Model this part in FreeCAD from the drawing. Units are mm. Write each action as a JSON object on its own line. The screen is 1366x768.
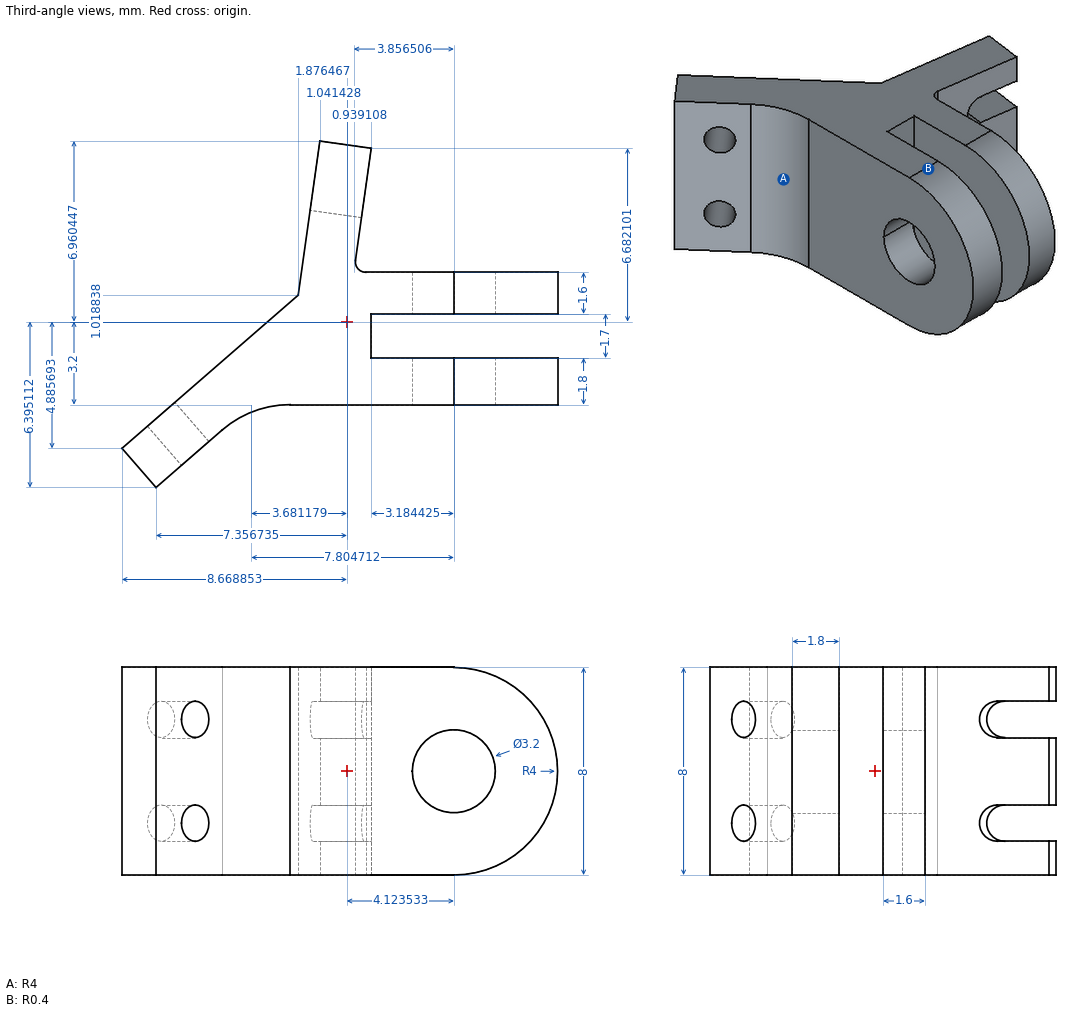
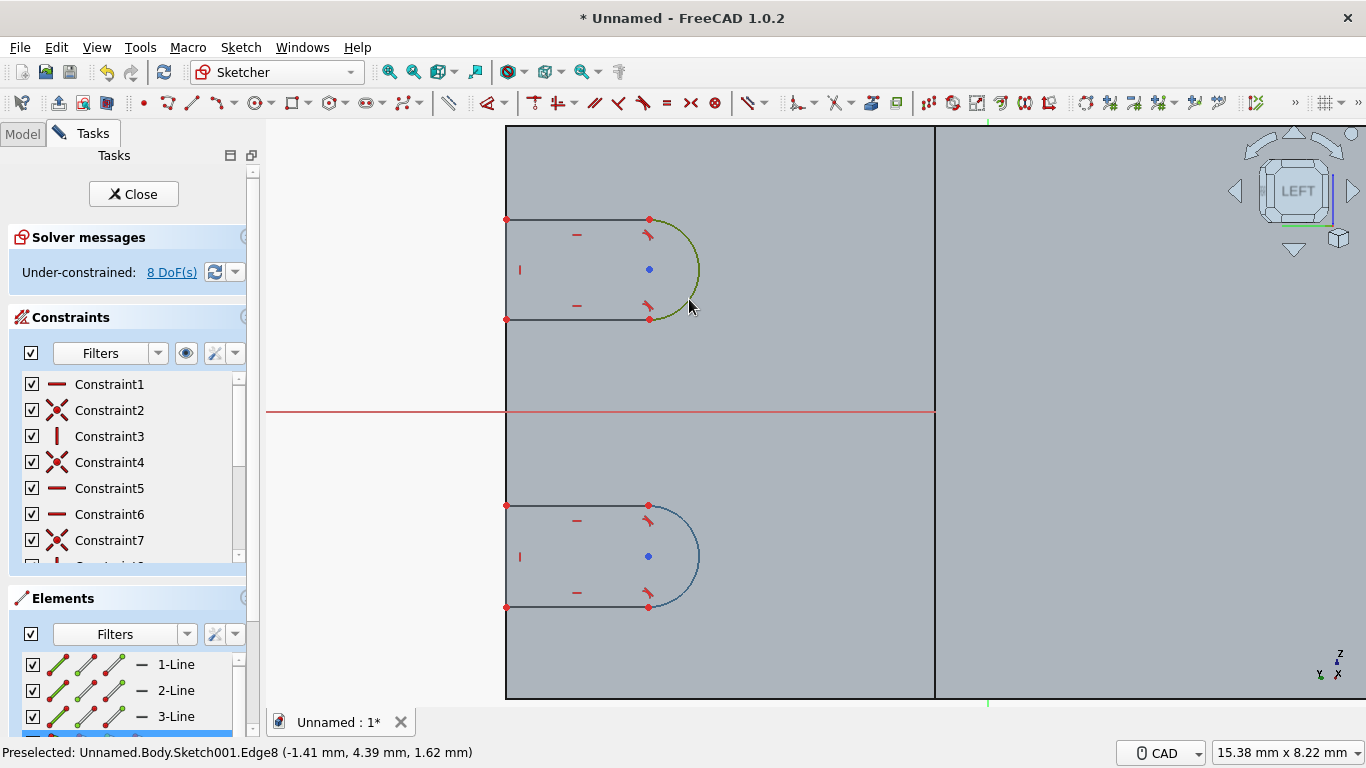
{"action": "left_click", "coordinate": [668, 104]}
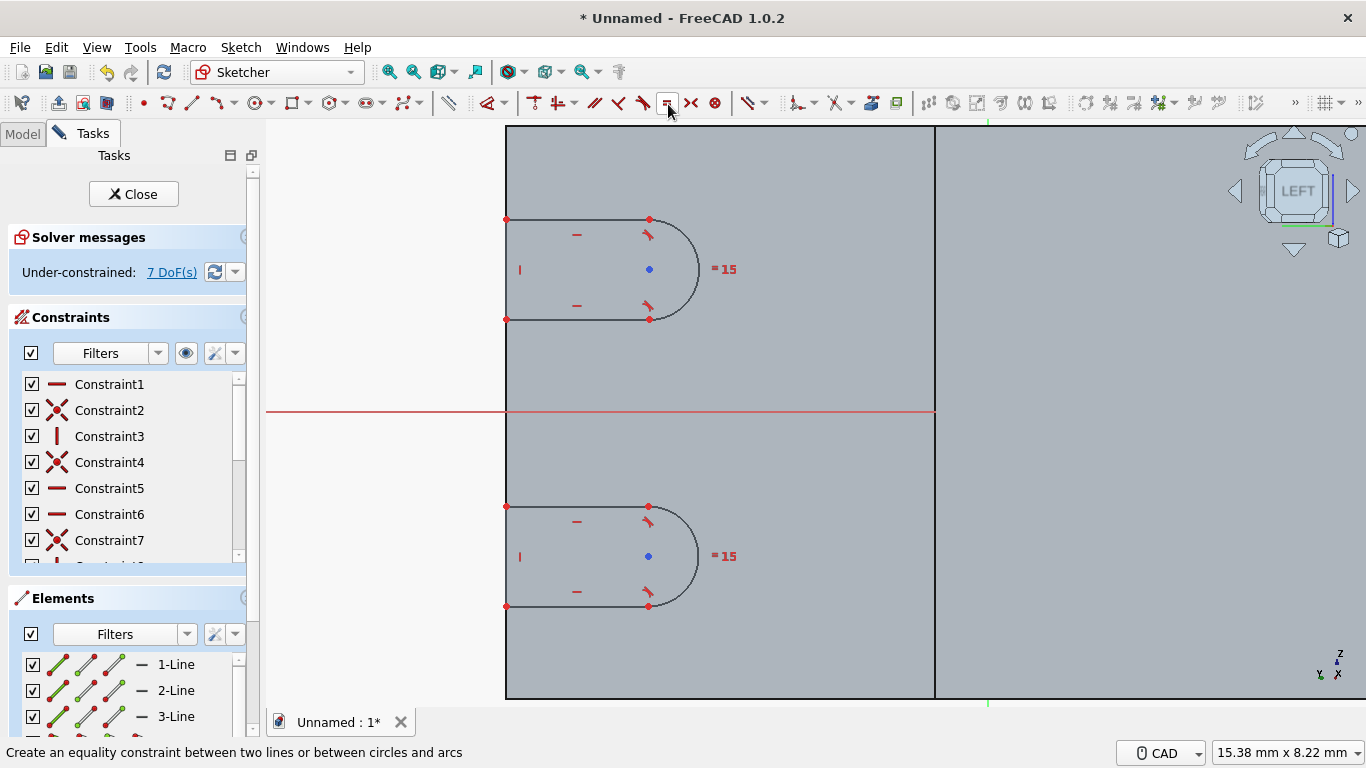
{"action": "left_click", "coordinate": [649, 557]}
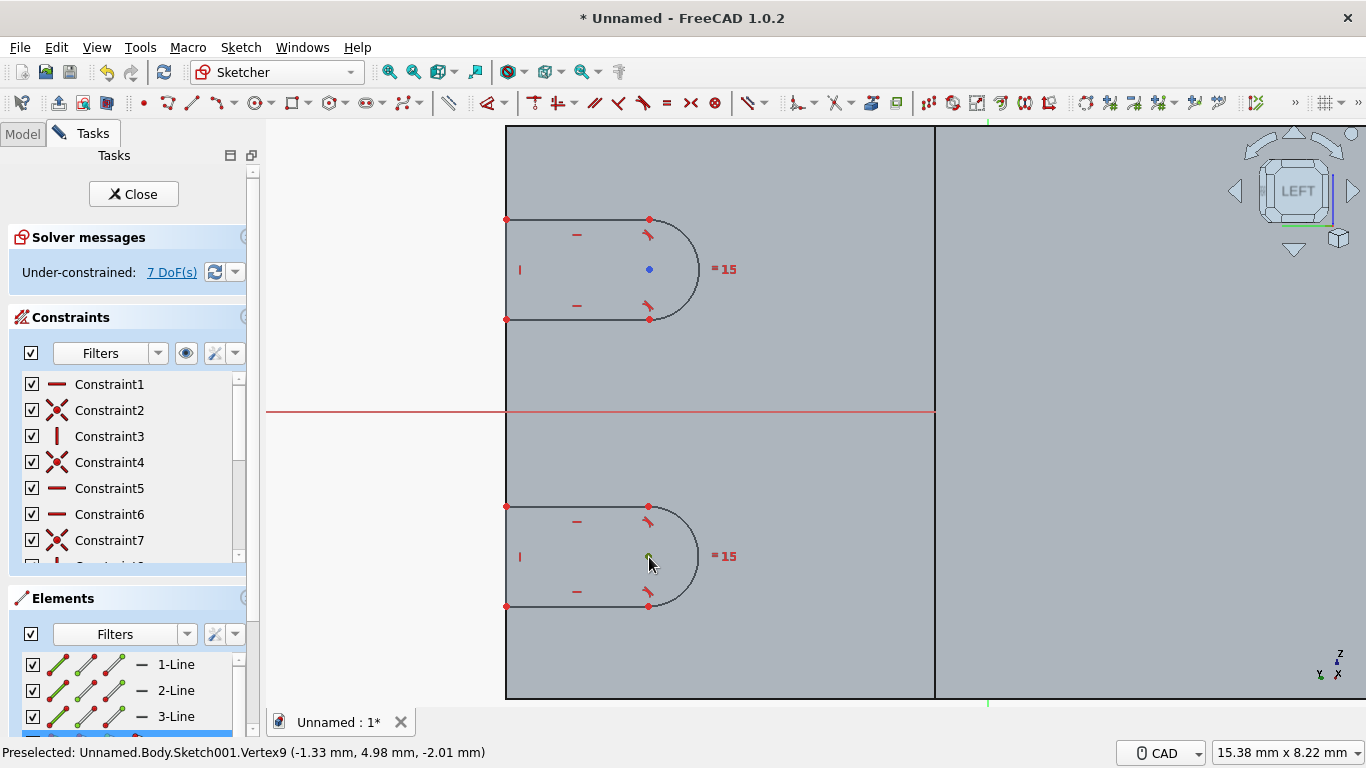
{"action": "left_click", "coordinate": [649, 270]}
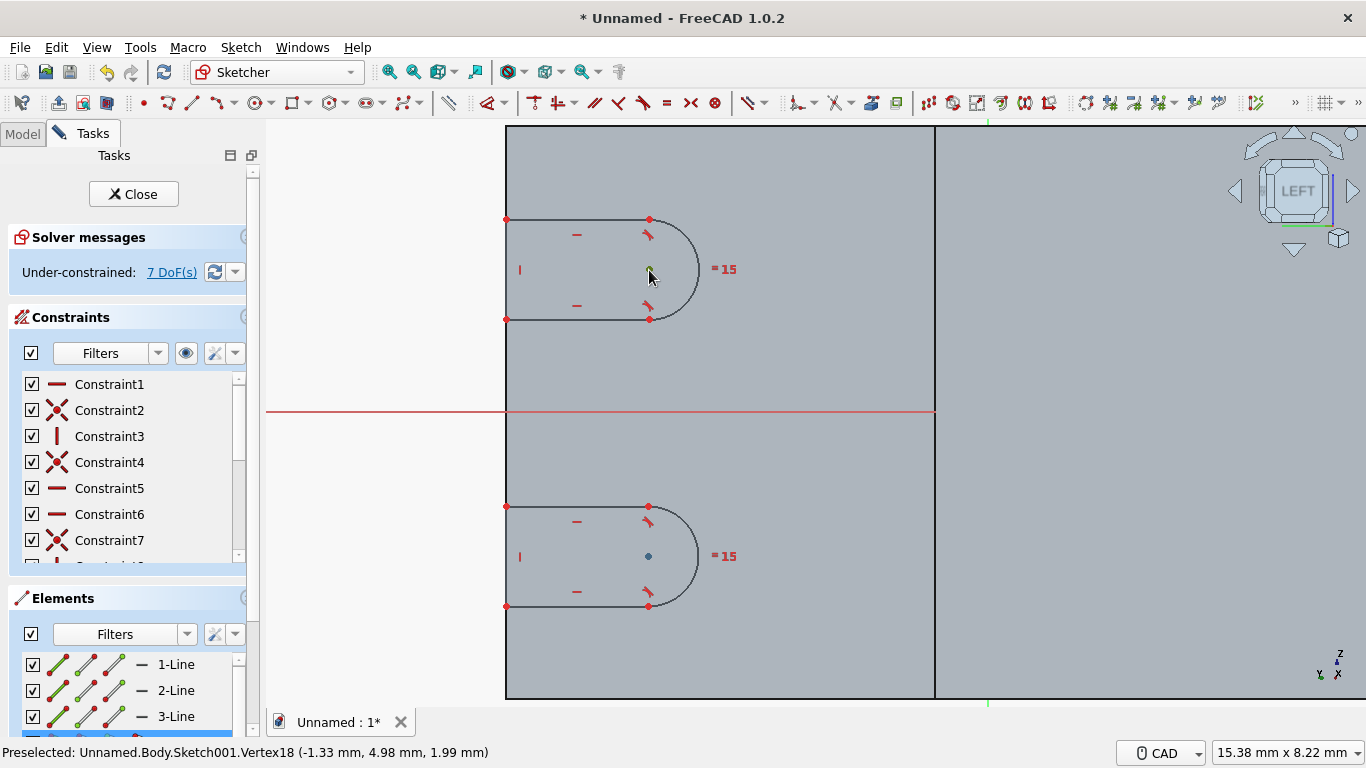
{"action": "left_click", "coordinate": [359, 412]}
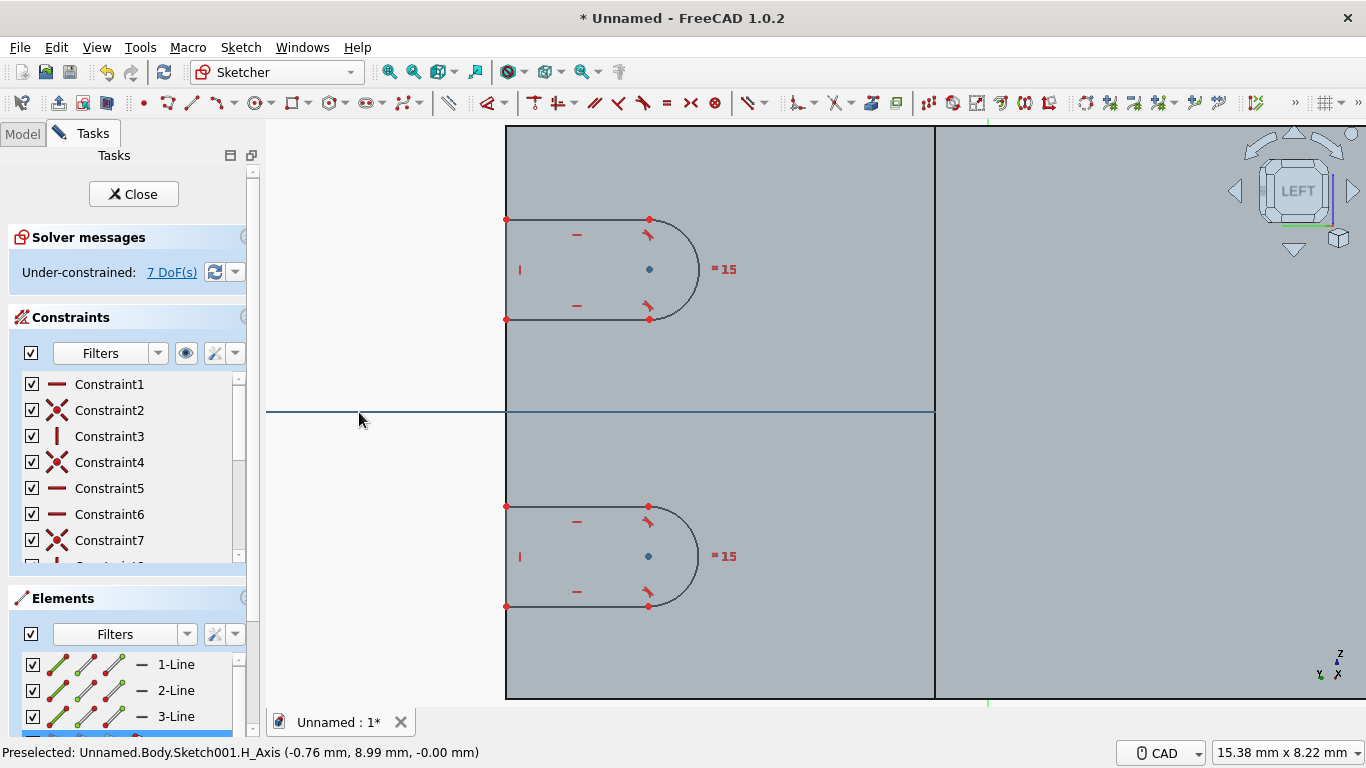
{"action": "left_click", "coordinate": [692, 104]}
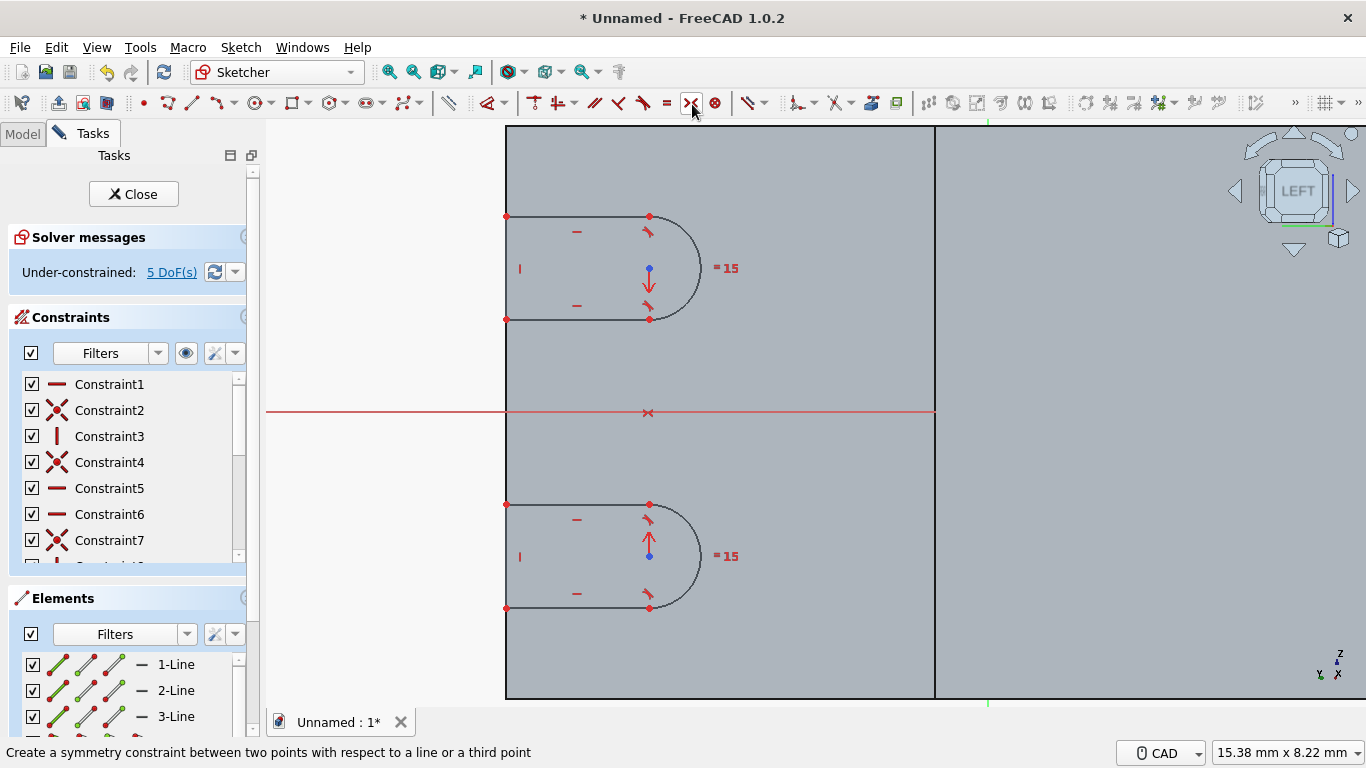
{"action": "left_click", "coordinate": [488, 104]}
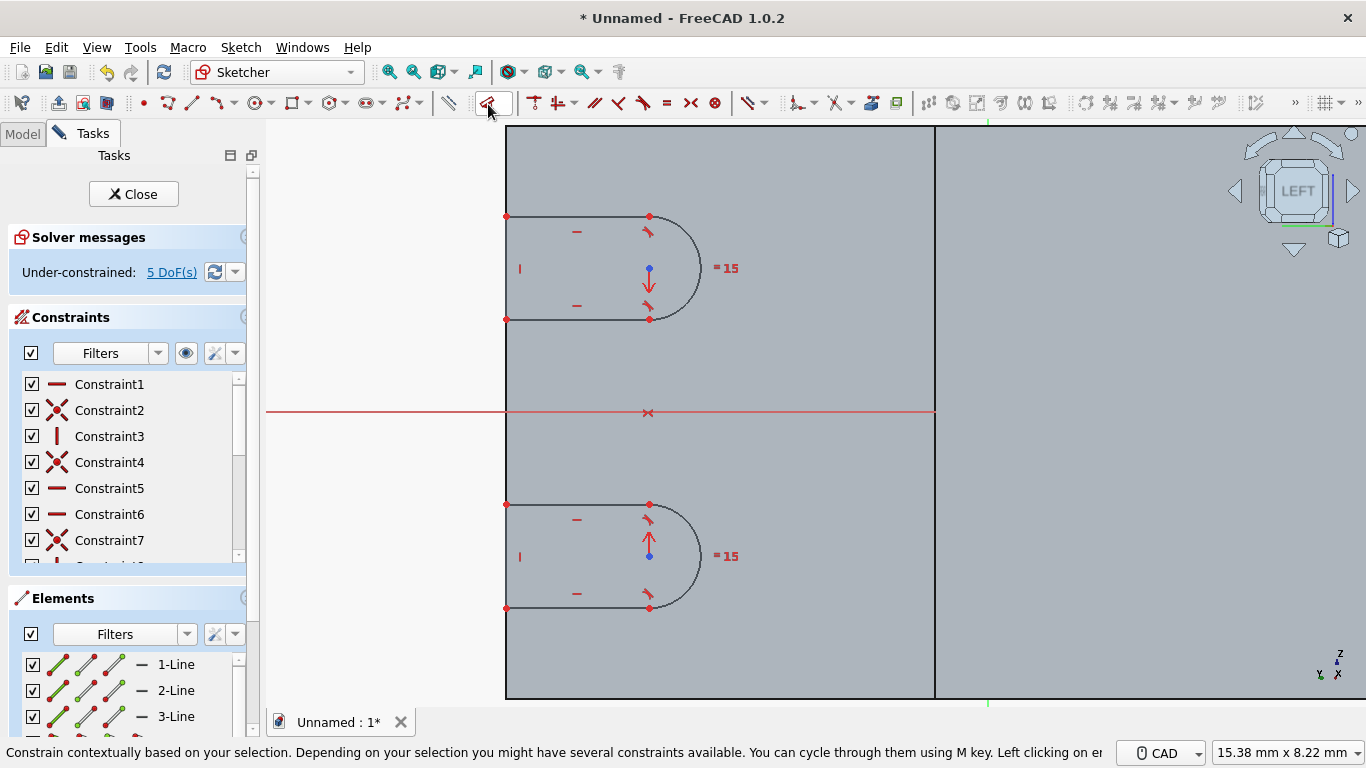
{"action": "left_click", "coordinate": [691, 587]}
{"action": "left_click", "coordinate": [717, 606]}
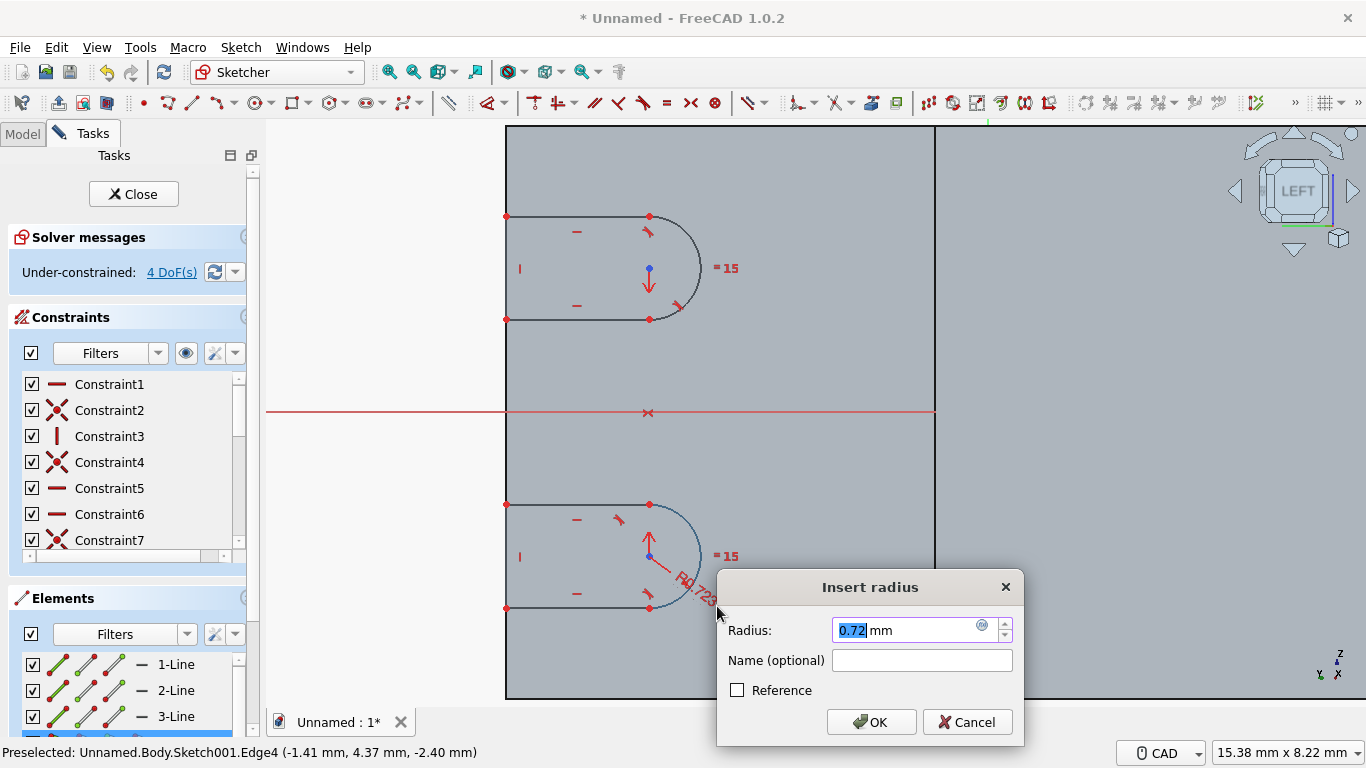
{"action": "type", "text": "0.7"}
{"action": "key", "text": "Return"}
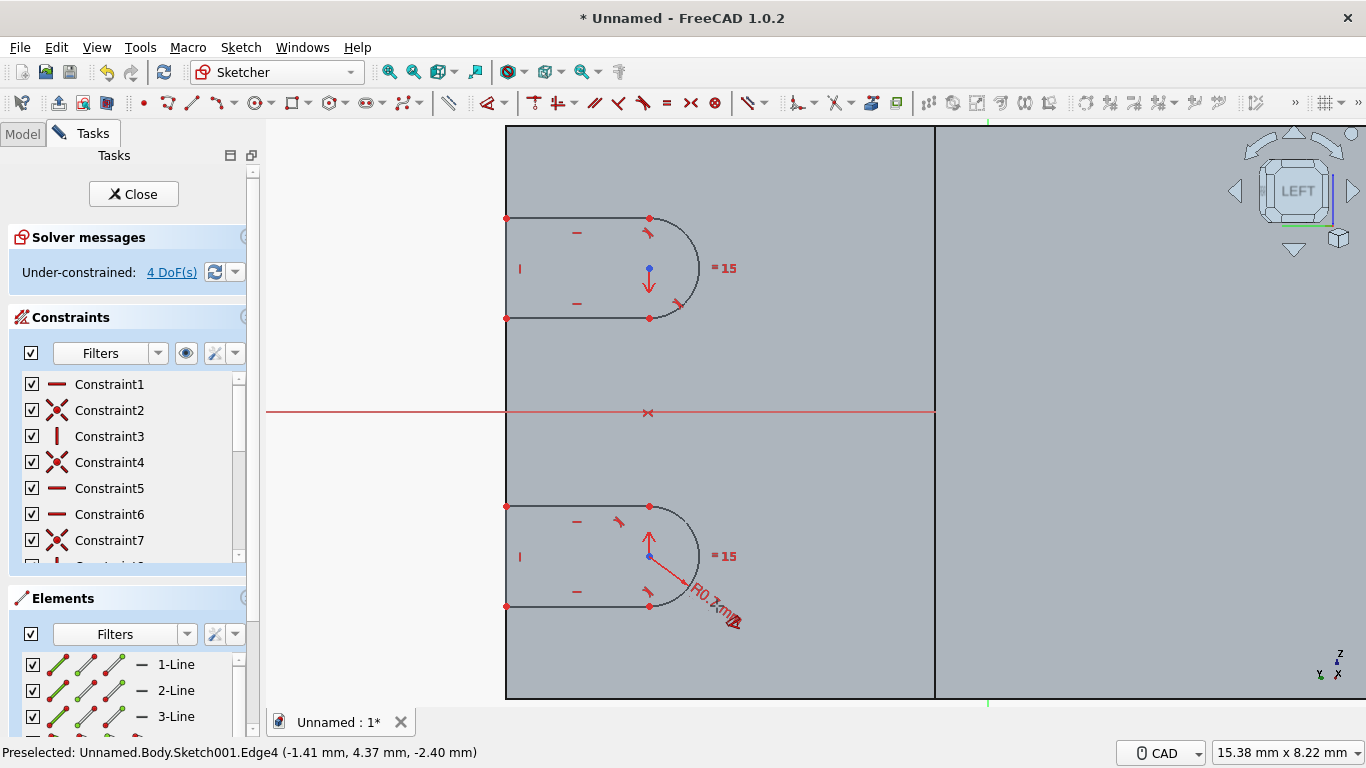
{"action": "left_click", "coordinate": [606, 506]}
{"action": "left_click", "coordinate": [578, 540]}